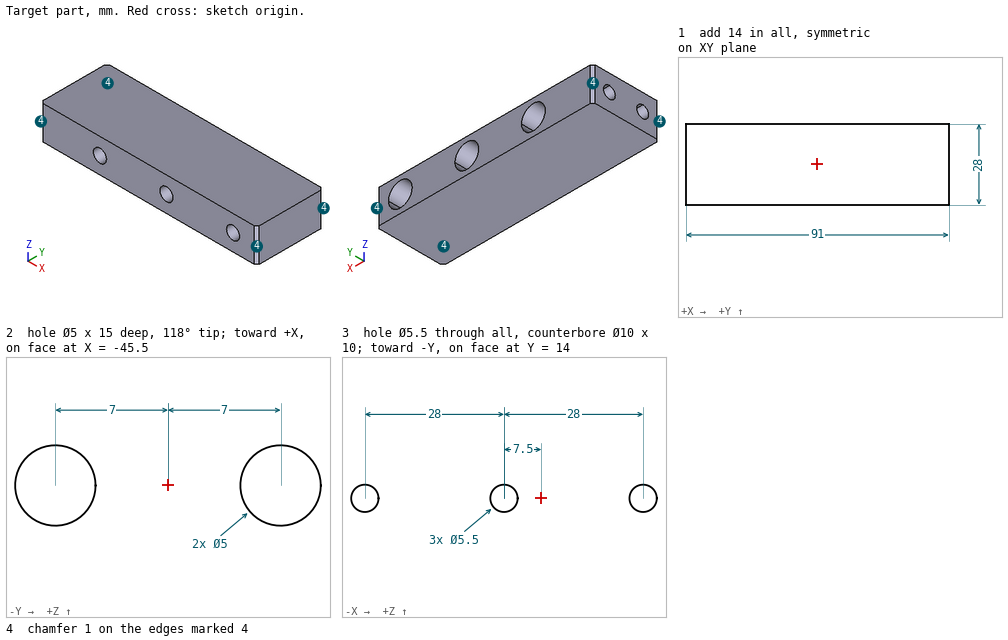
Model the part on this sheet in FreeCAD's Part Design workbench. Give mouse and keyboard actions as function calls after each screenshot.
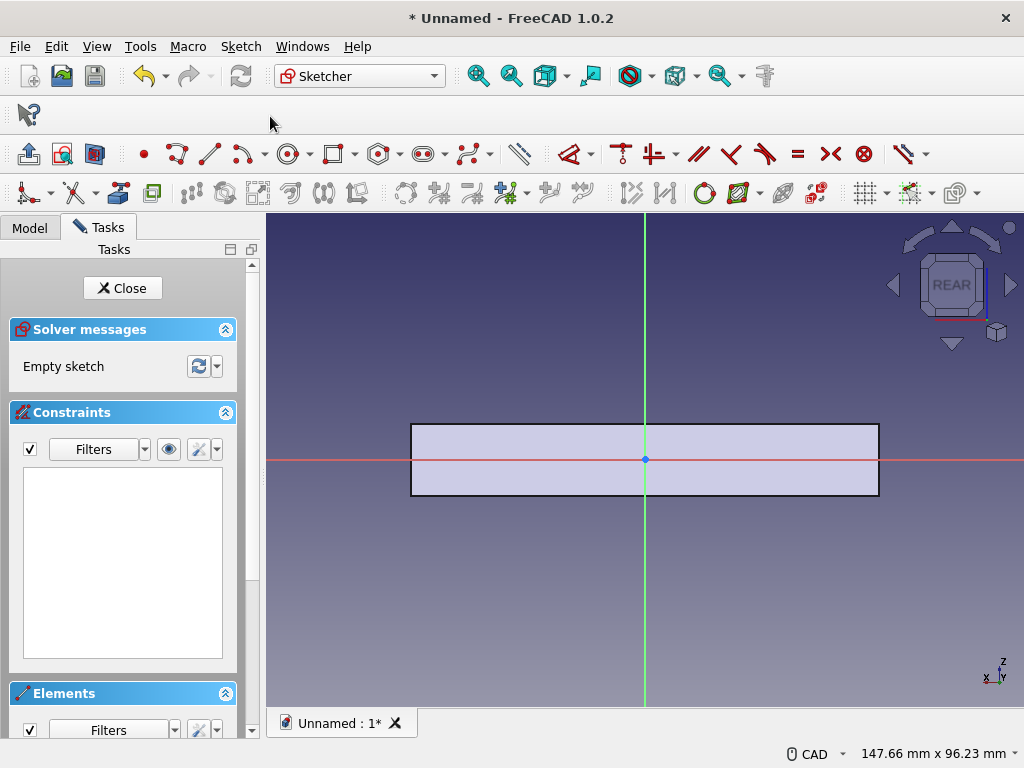
click(288, 154)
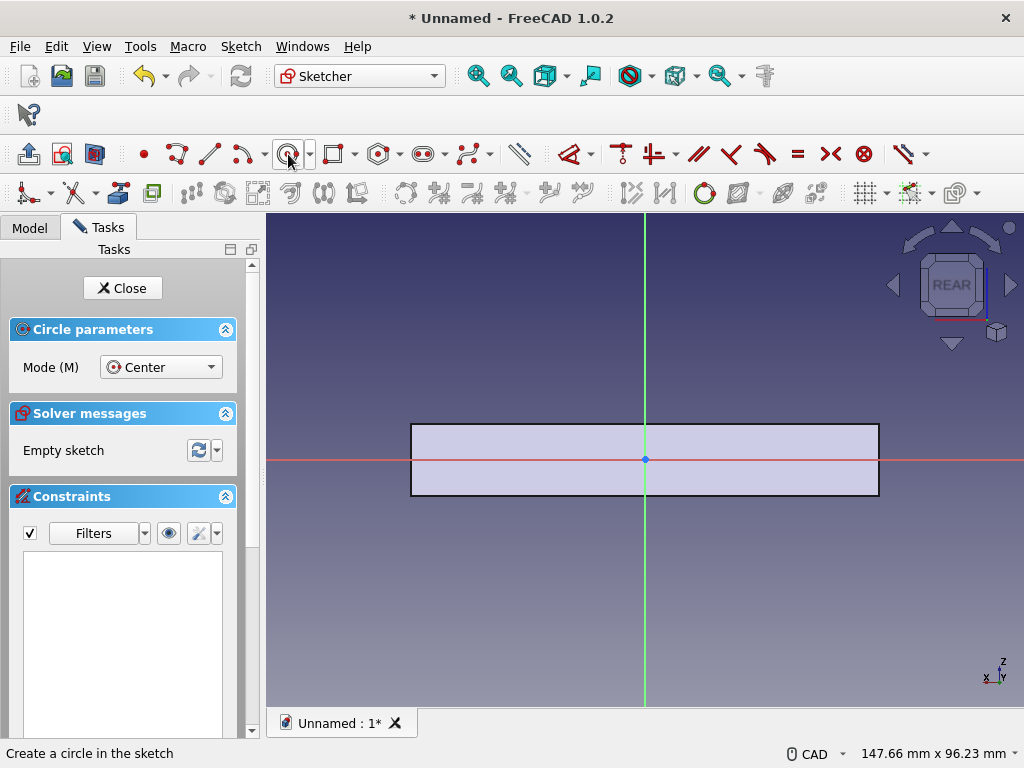
scroll(607, 460, up, 3)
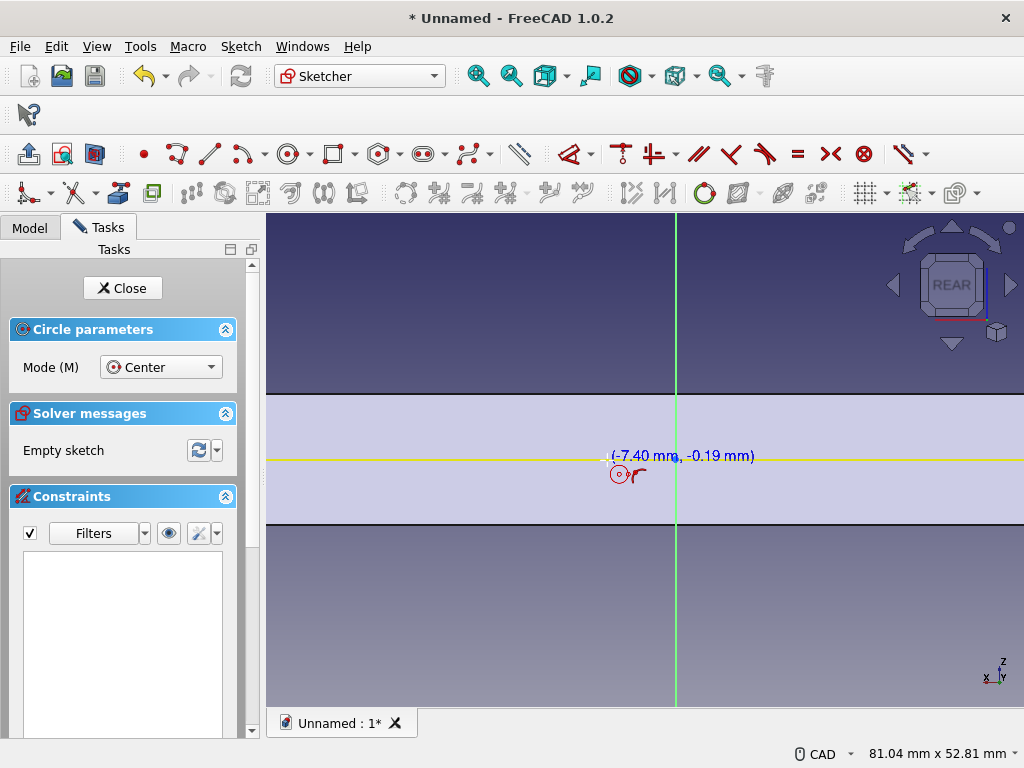
click(606, 460)
move(624, 441)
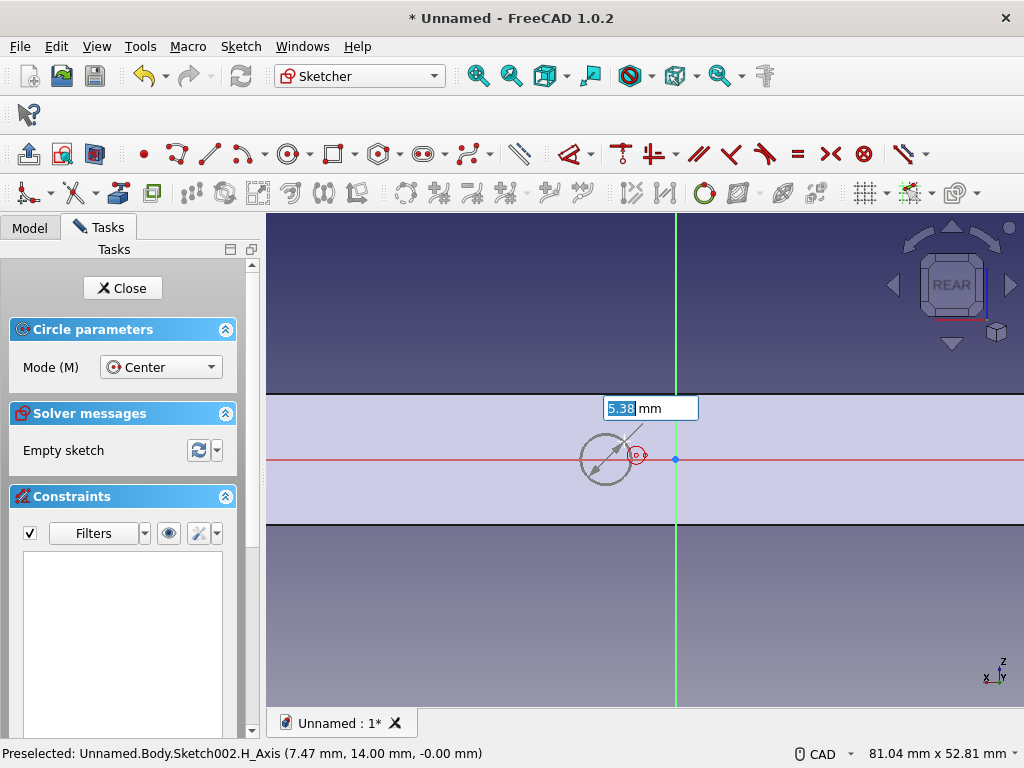
text(5.5)
key(Return)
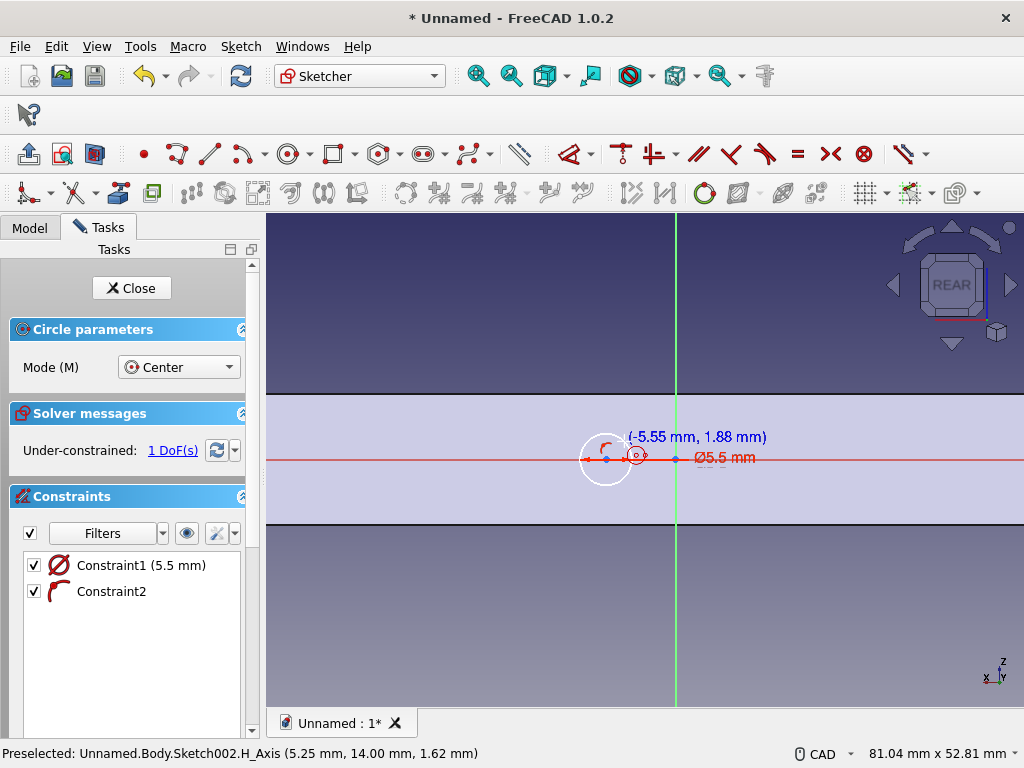
scroll(517, 461, down, 2)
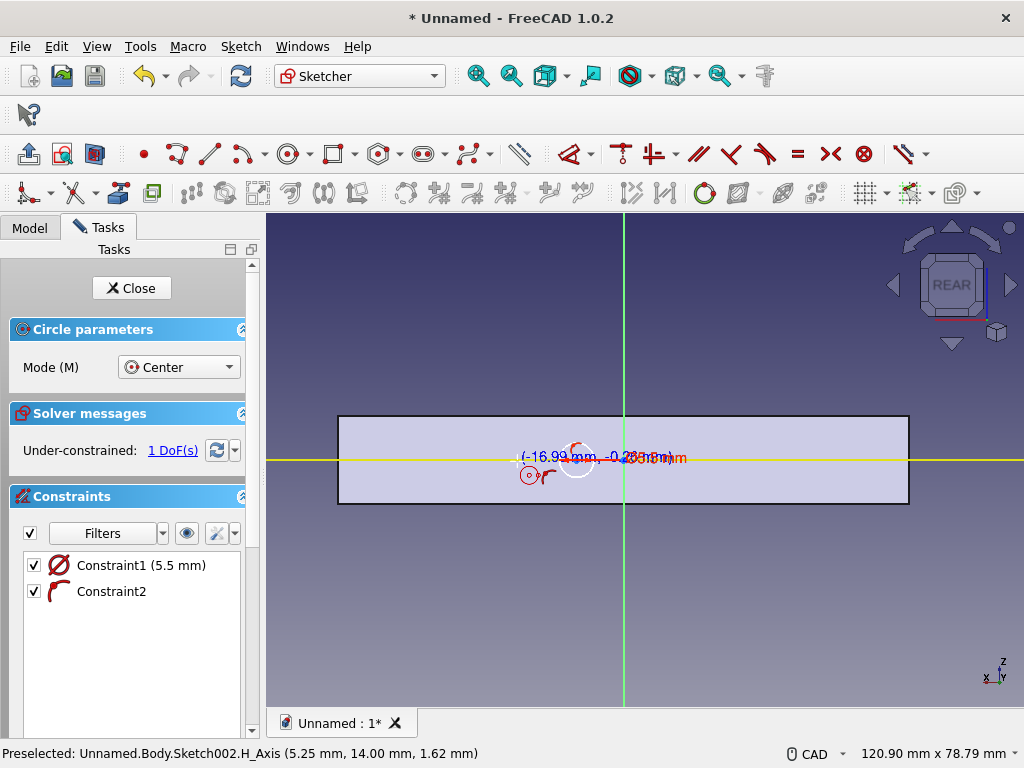
scroll(752, 460, up, 2)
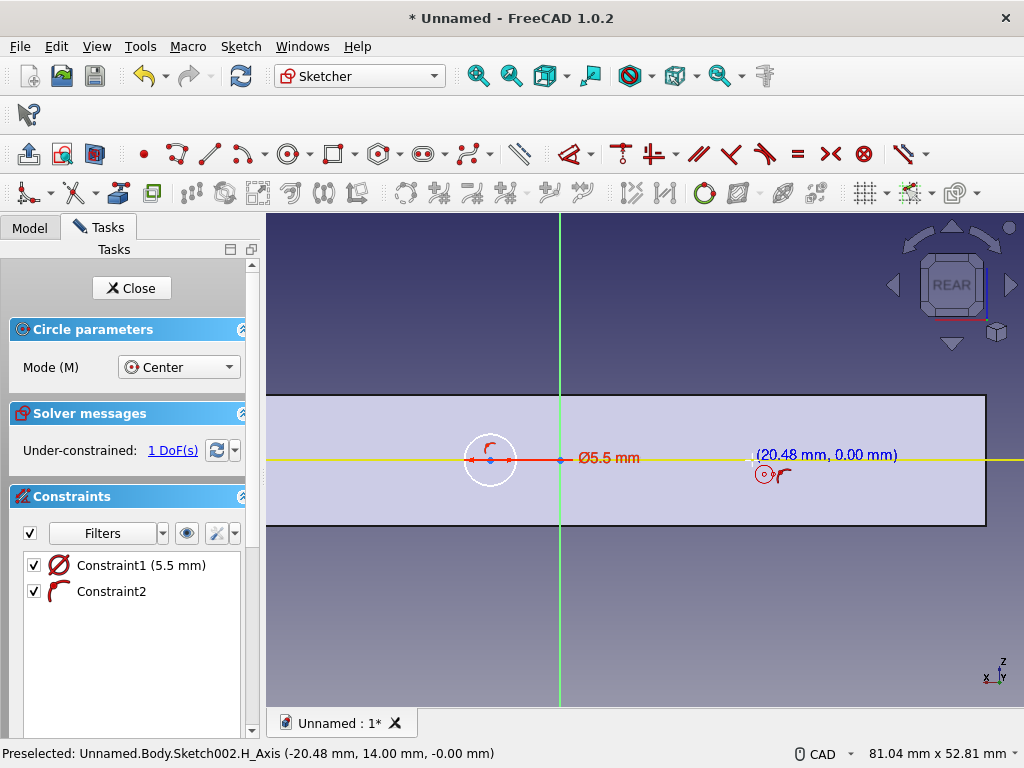
click(752, 460)
move(770, 442)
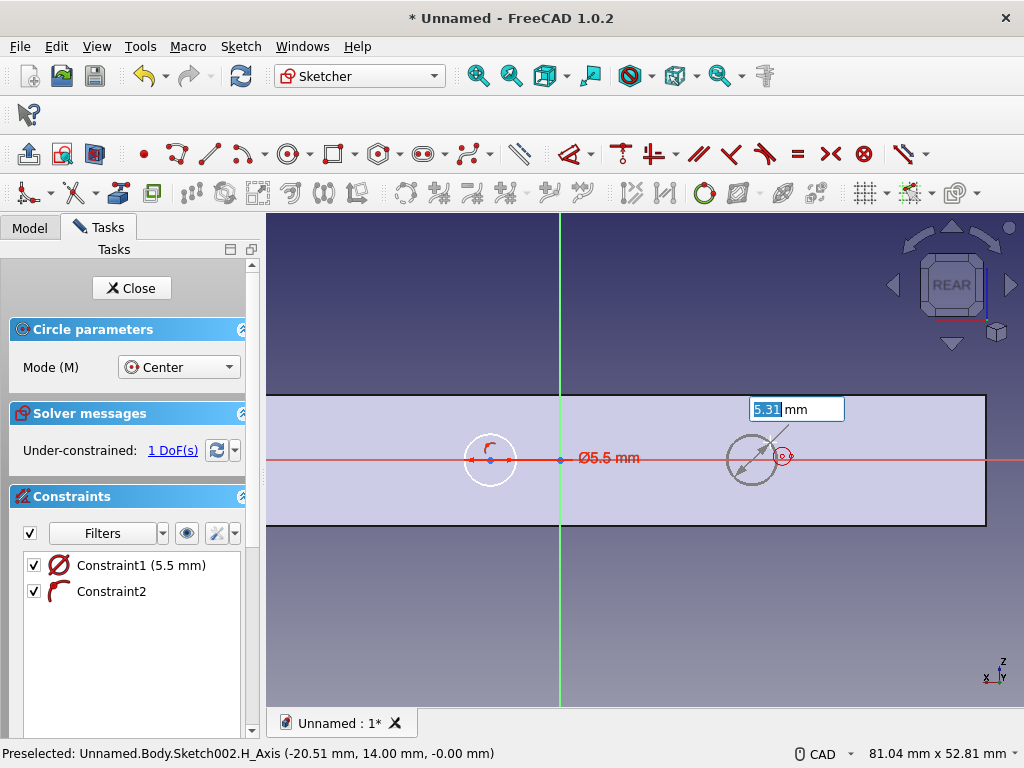
text(5.5)
key(Return)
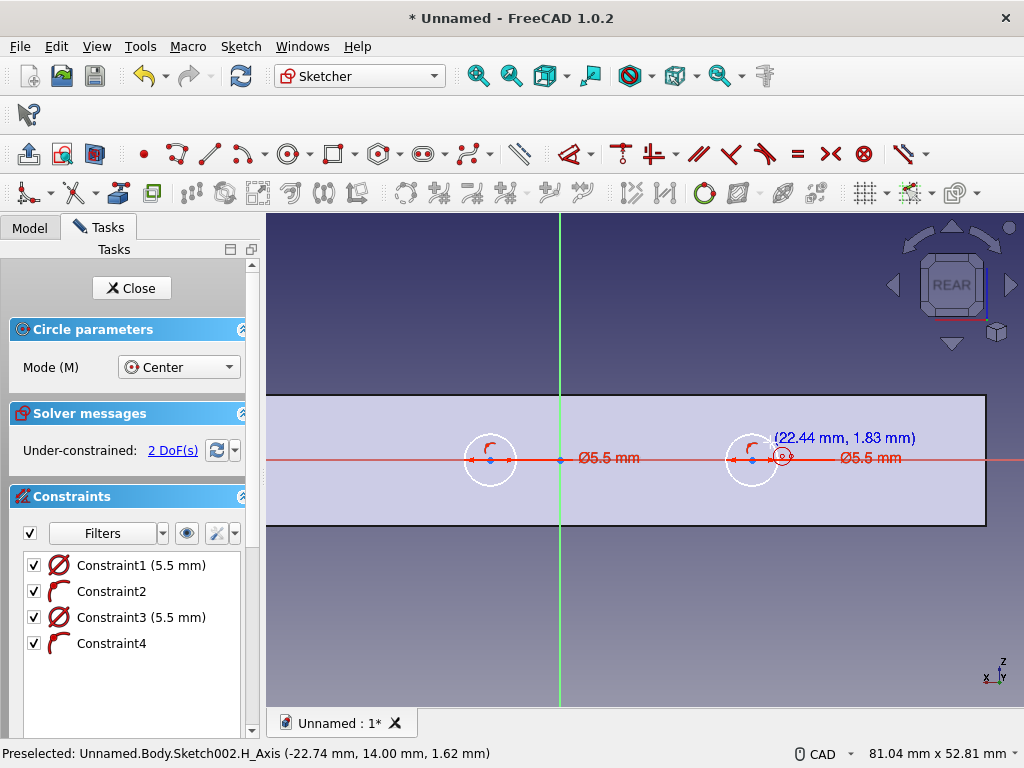
scroll(752, 460, down, 2)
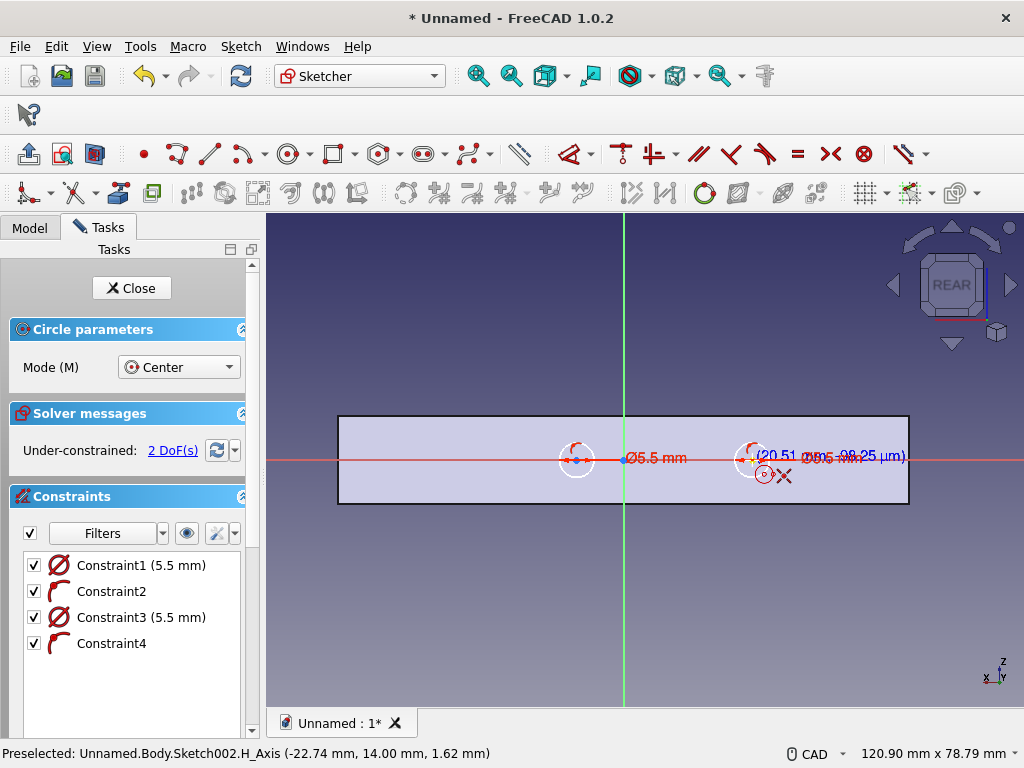
scroll(401, 460, up, 2)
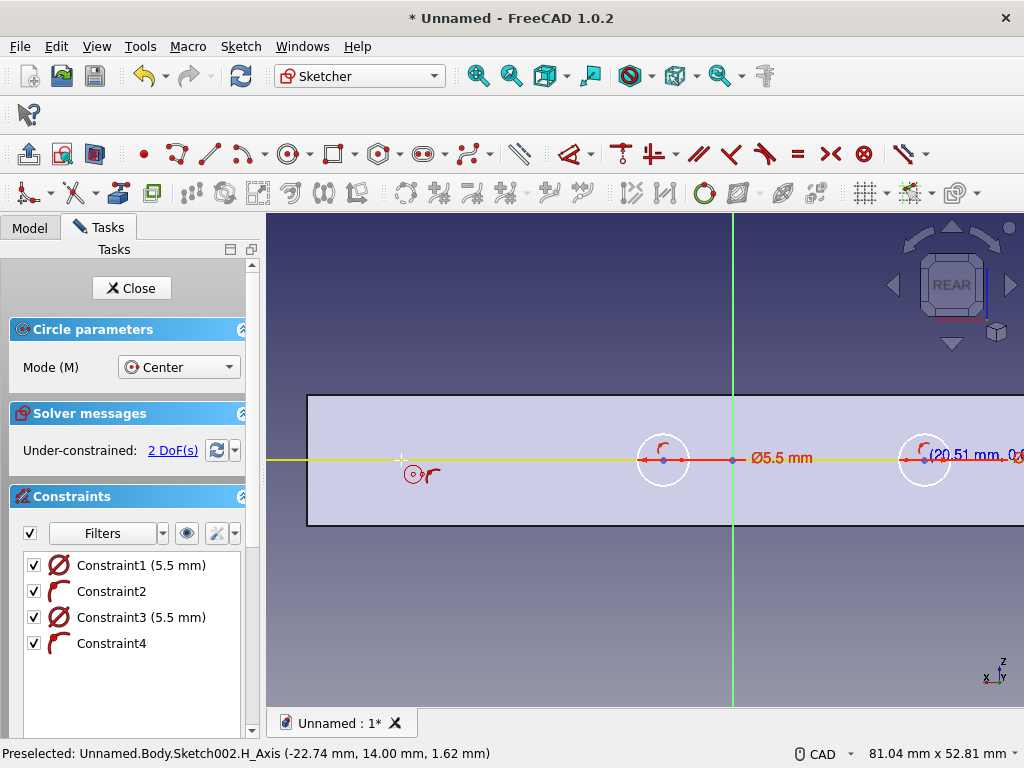
click(401, 460)
move(419, 442)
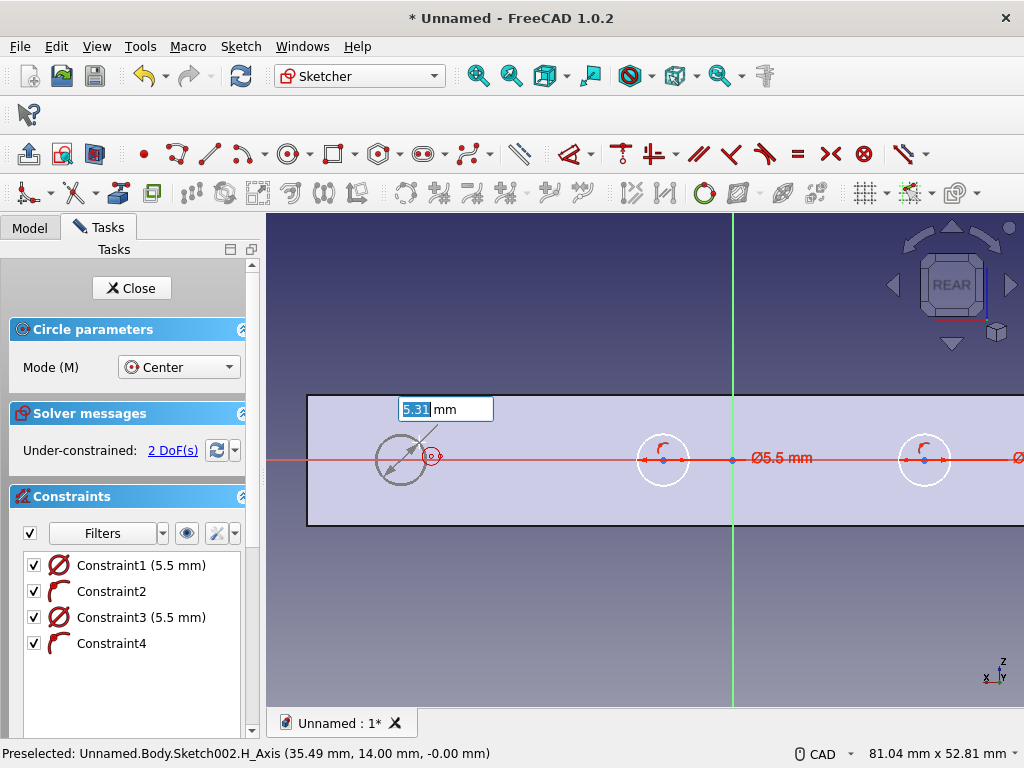
text(5.5)
key(Return)
key(Escape)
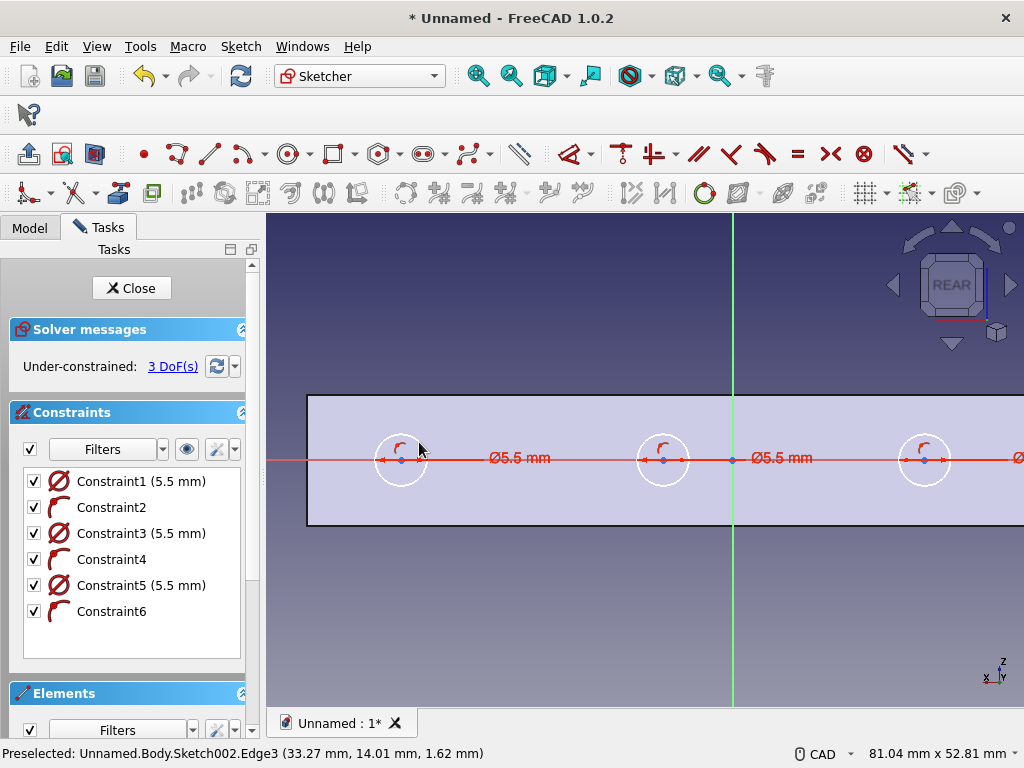
key(d)